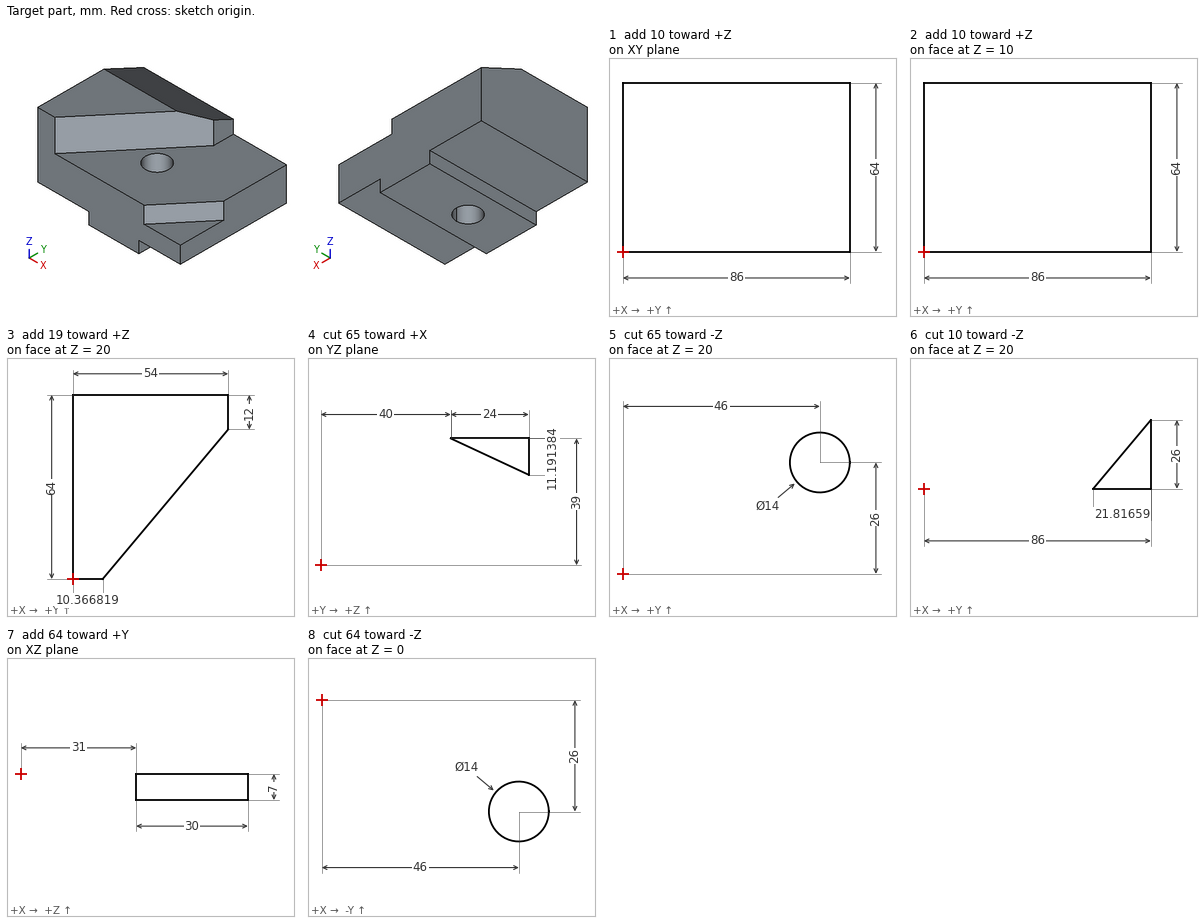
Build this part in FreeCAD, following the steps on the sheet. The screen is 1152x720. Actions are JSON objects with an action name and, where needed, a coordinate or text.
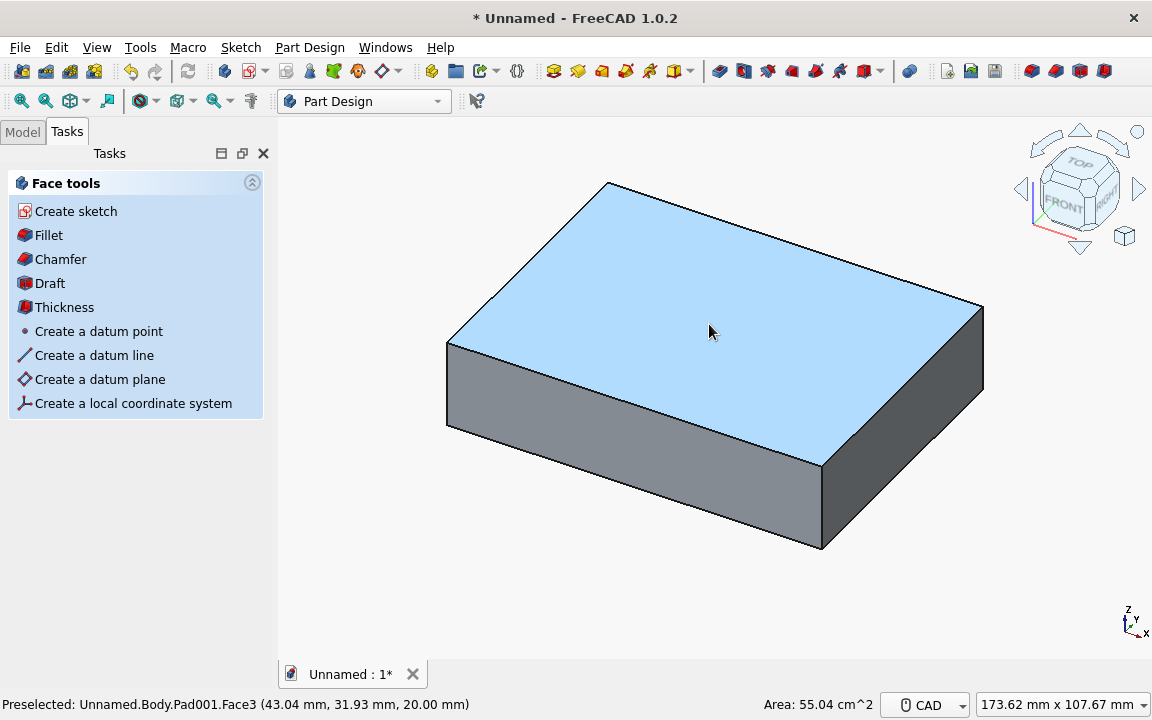
{"action": "left_click", "coordinate": [250, 72]}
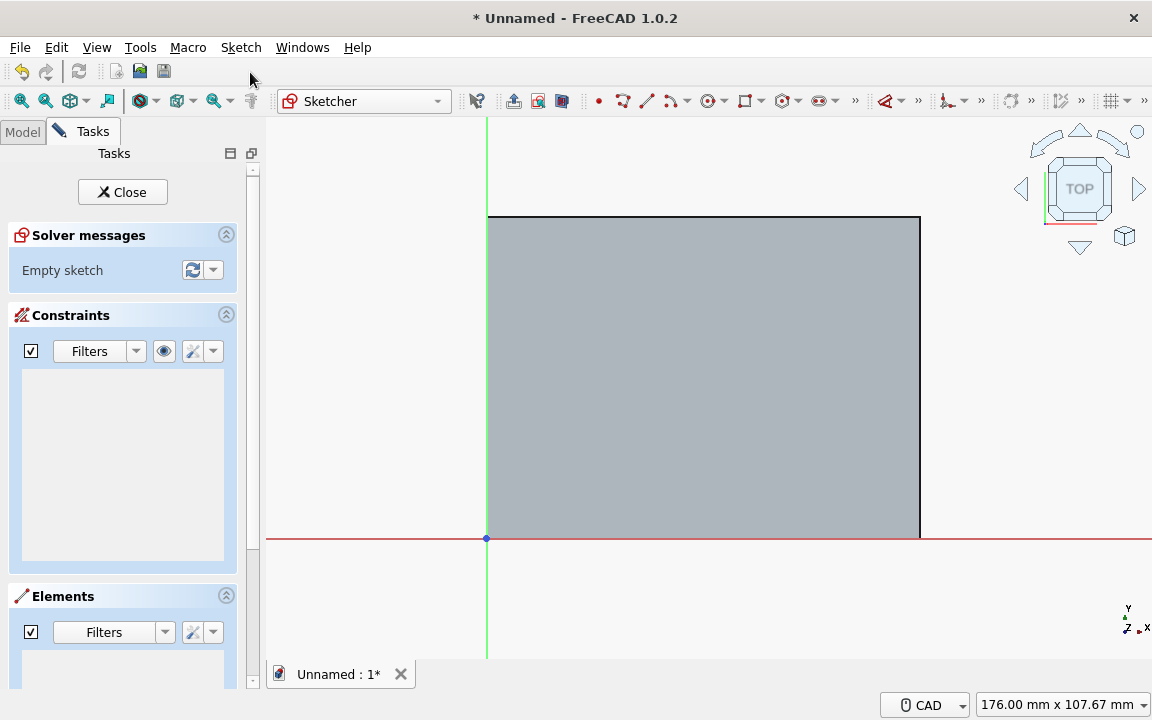
{"action": "left_click", "coordinate": [624, 102]}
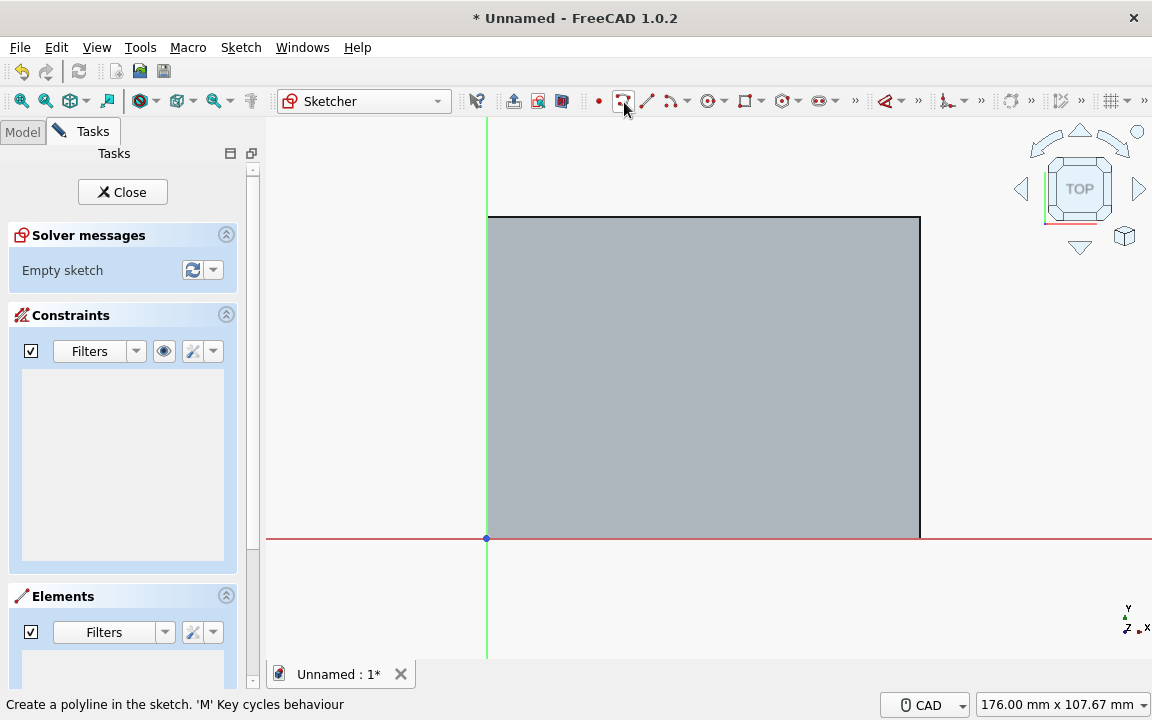
{"action": "left_click", "coordinate": [487, 539]}
{"action": "left_click", "coordinate": [539, 530]}
{"action": "left_click", "coordinate": [758, 277]}
{"action": "left_click", "coordinate": [758, 217]}
{"action": "left_click", "coordinate": [496, 217]}
{"action": "left_click", "coordinate": [487, 539]}
{"action": "key", "text": "Escape"}
{"action": "key", "text": "Escape"}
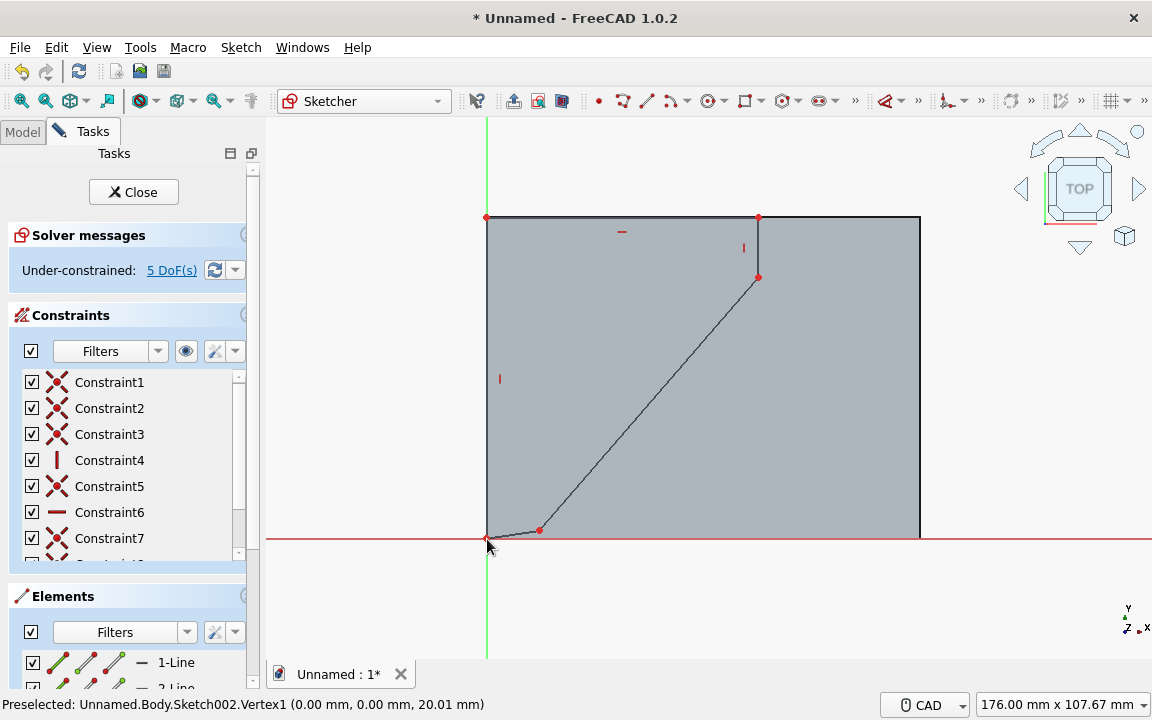
{"action": "left_click", "coordinate": [502, 536]}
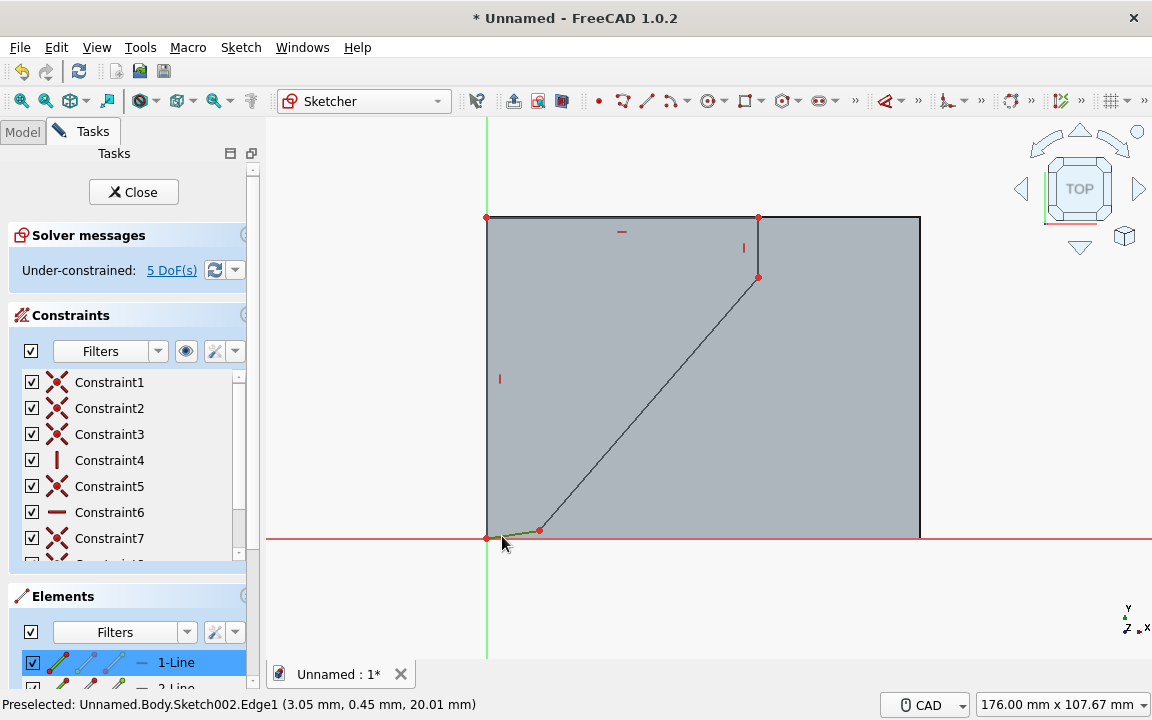
{"action": "key", "text": "h"}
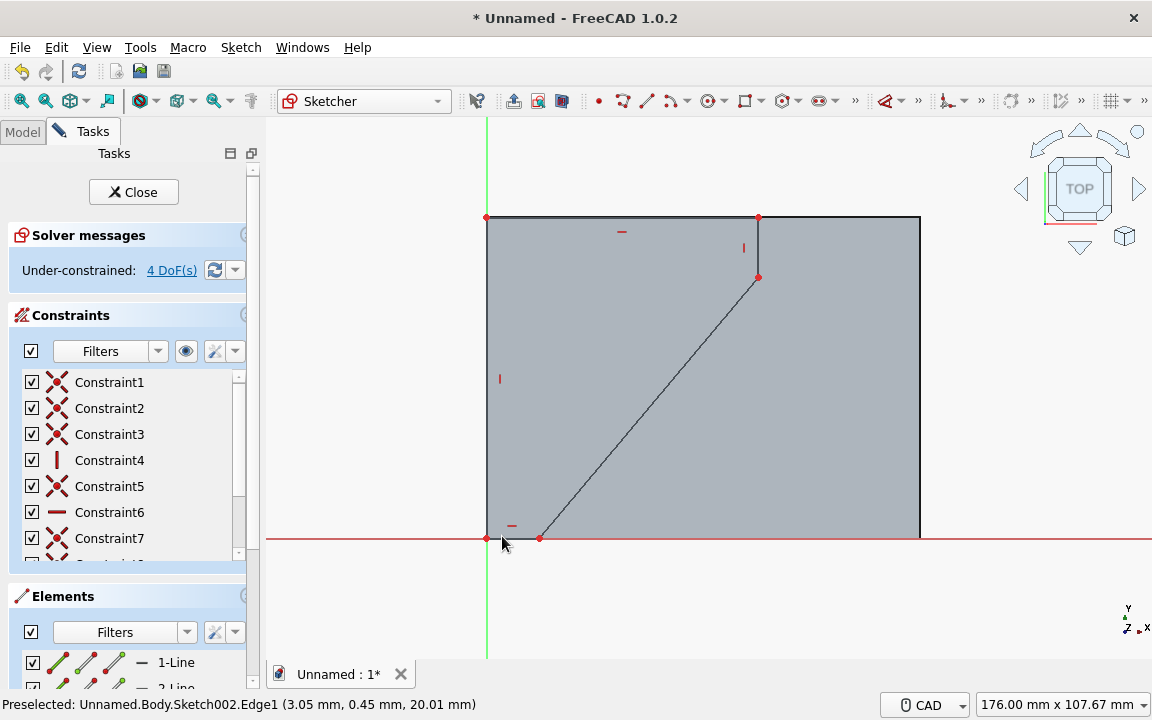
{"action": "left_click", "coordinate": [886, 102]}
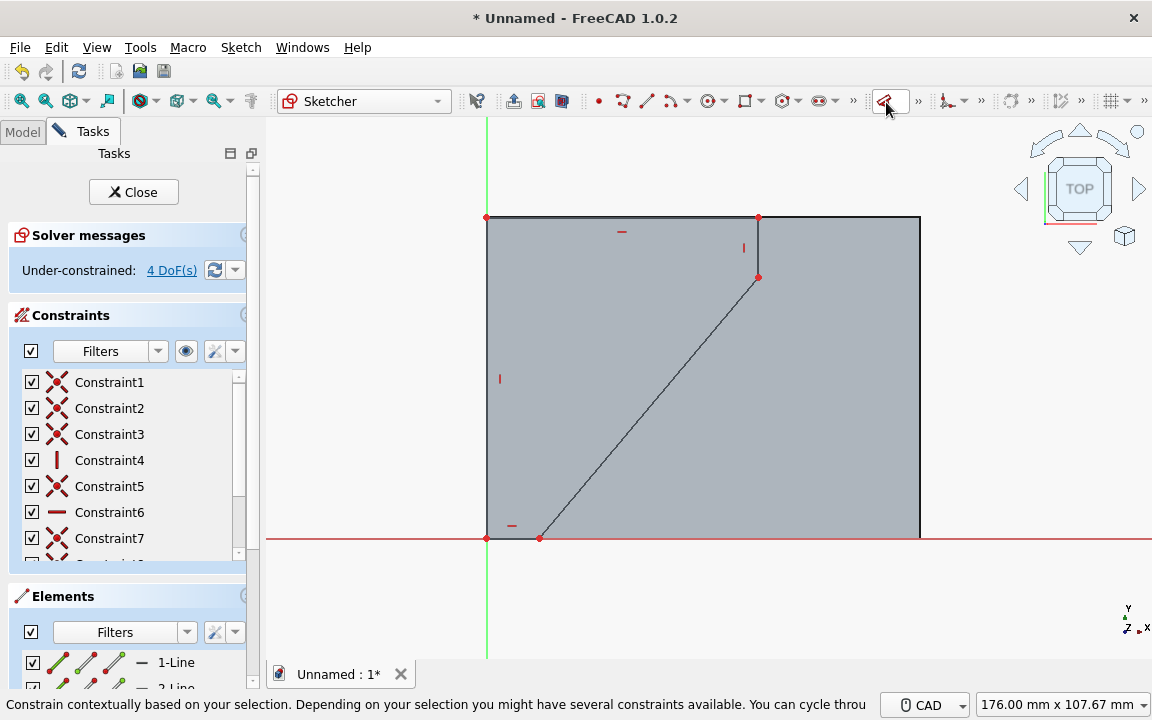
{"action": "left_click", "coordinate": [758, 260]}
{"action": "left_click", "coordinate": [792, 248]}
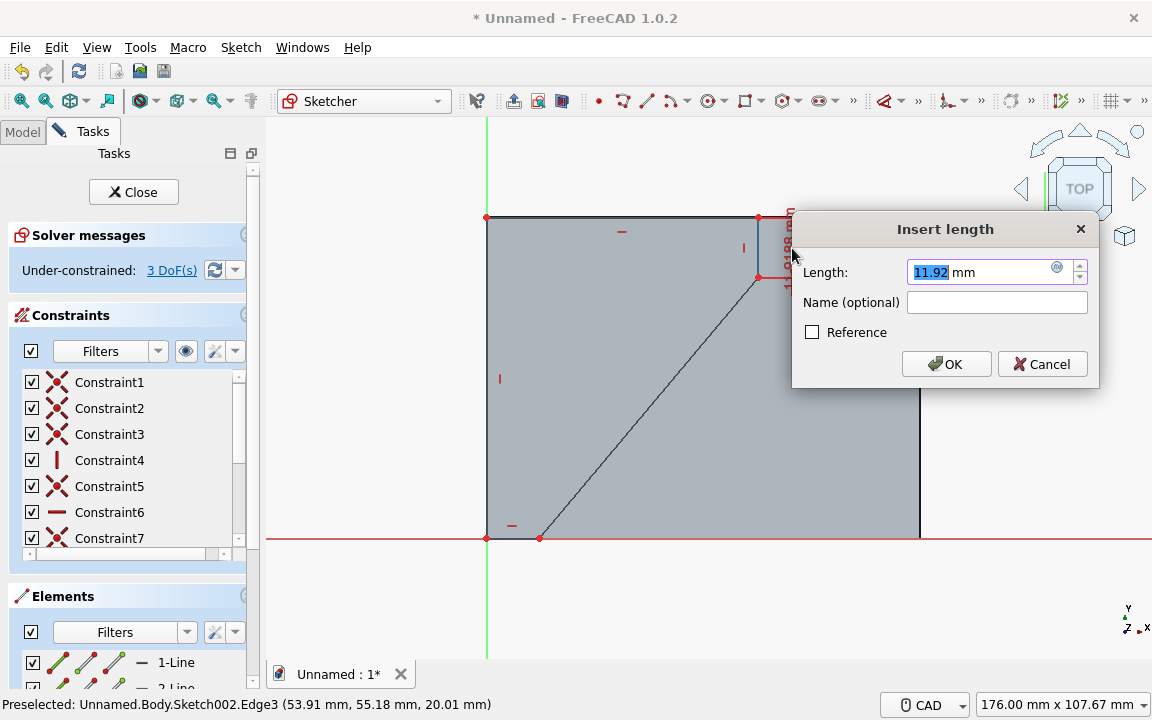
{"action": "type", "text": "12"}
{"action": "key", "text": "Return"}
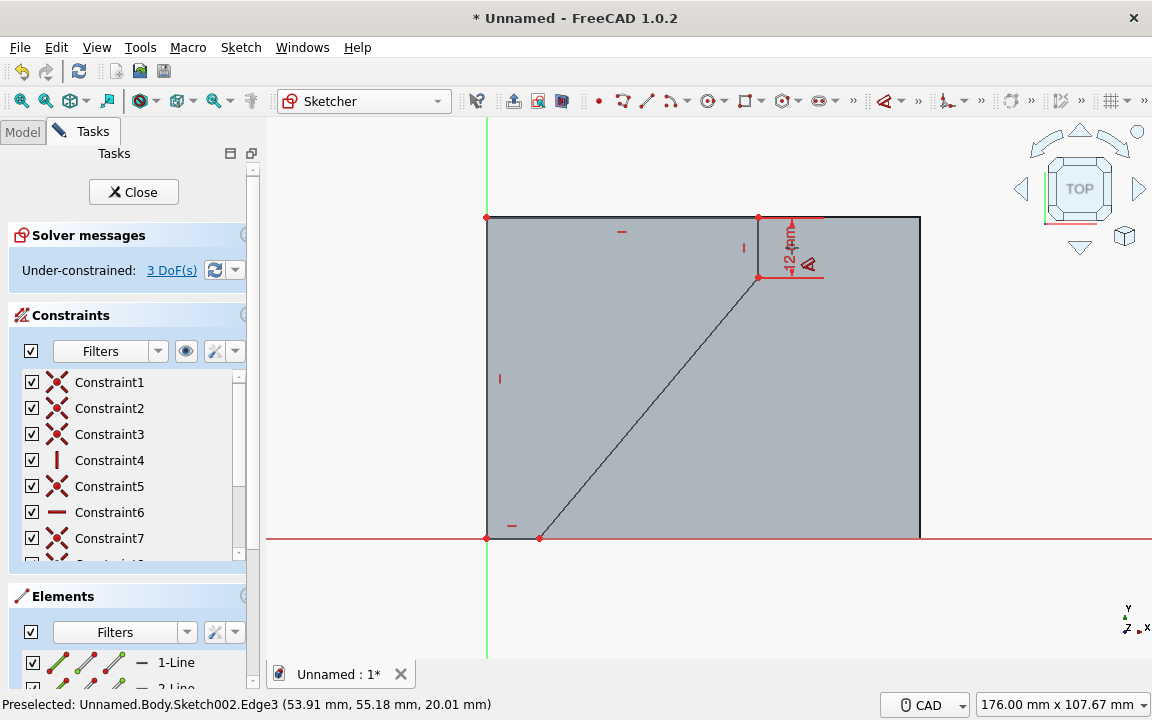
{"action": "left_click", "coordinate": [677, 218]}
{"action": "left_click", "coordinate": [622, 184]}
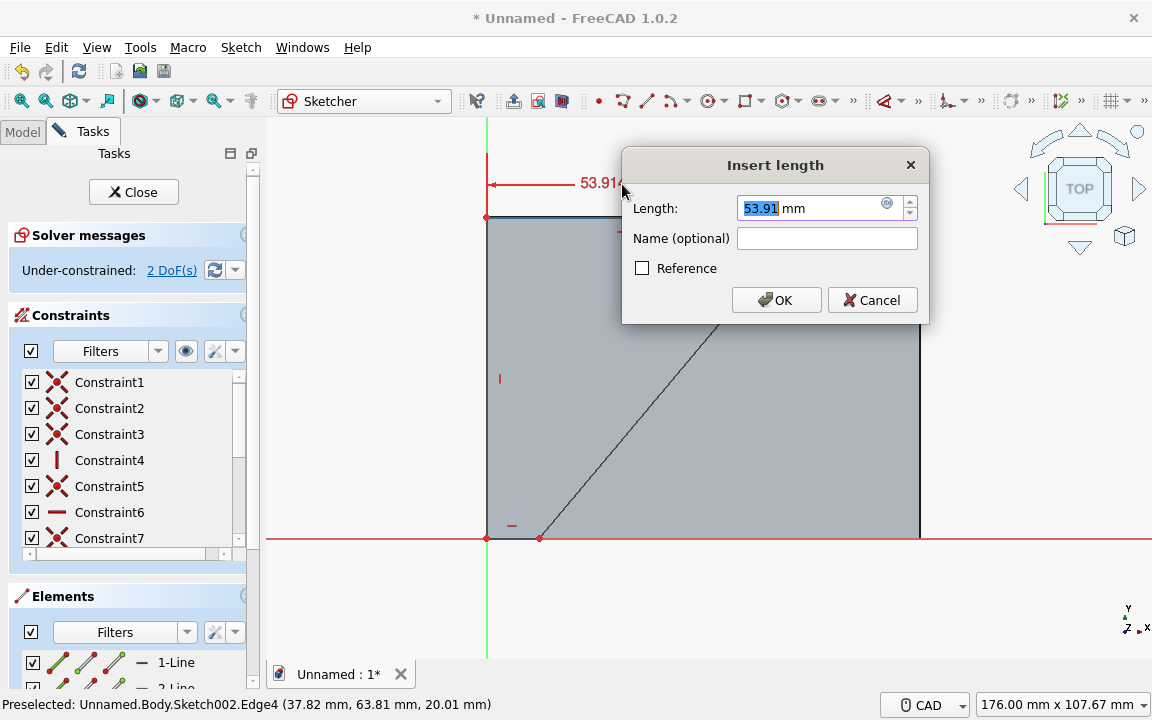
{"action": "type", "text": "54"}
{"action": "key", "text": "Return"}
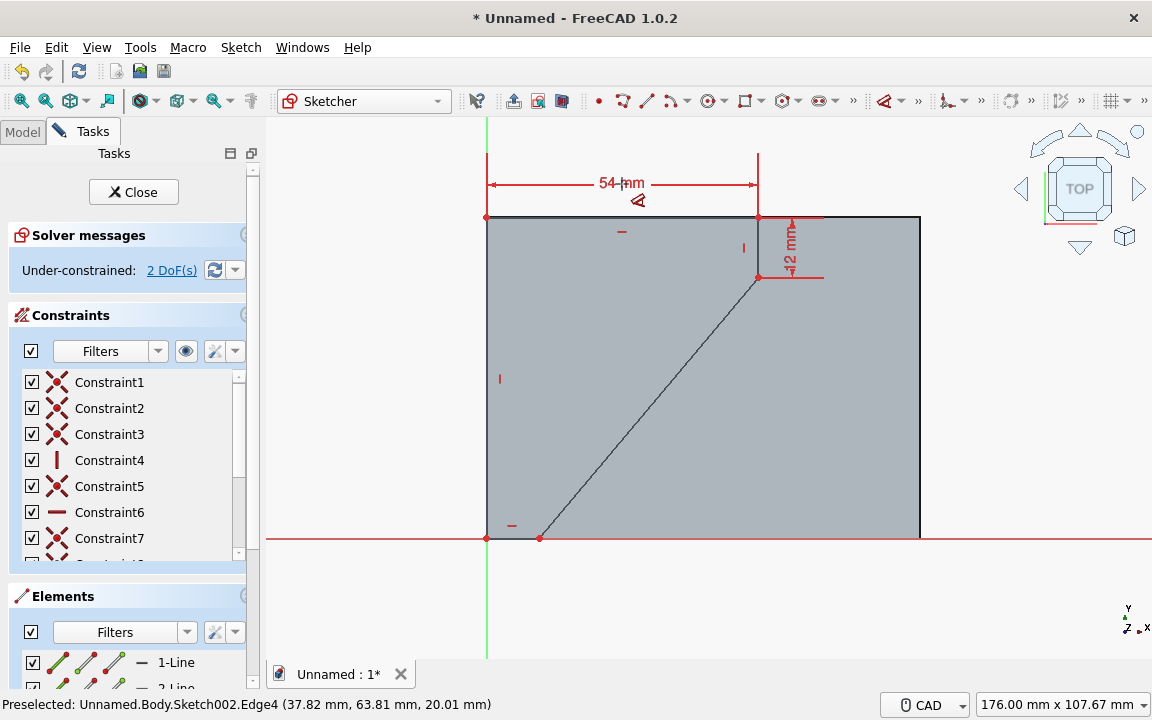
{"action": "left_click", "coordinate": [487, 314]}
{"action": "left_click", "coordinate": [453, 378]}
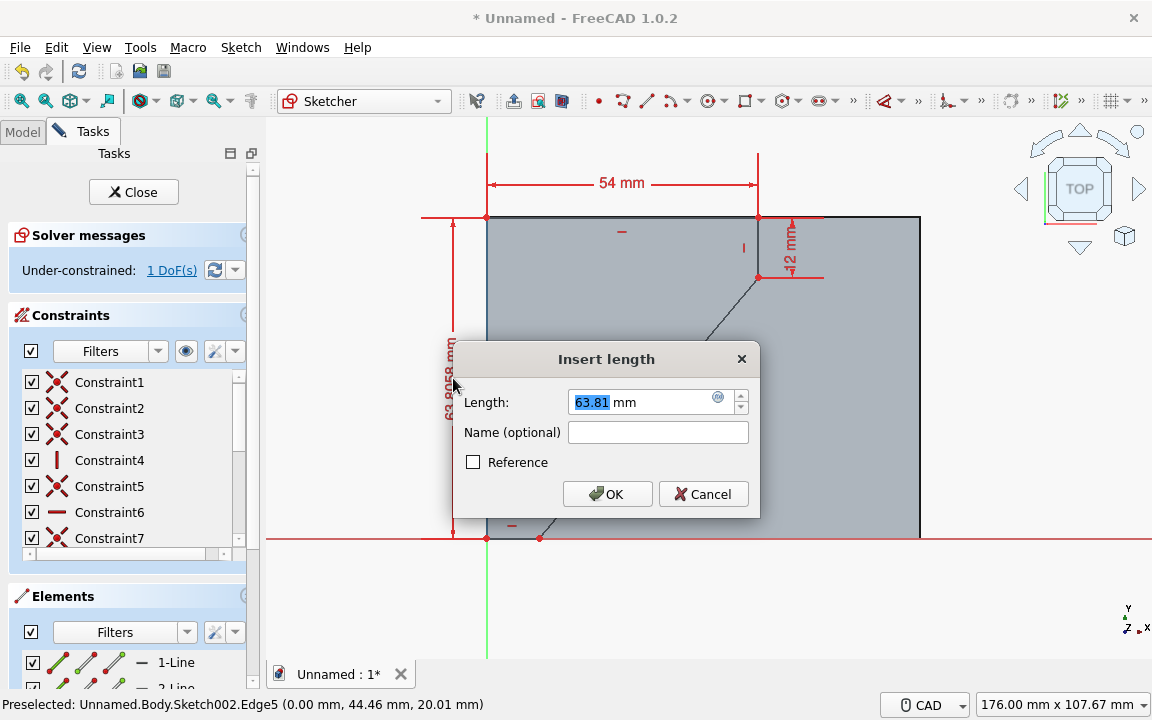
{"action": "type", "text": "64"}
{"action": "key", "text": "Return"}